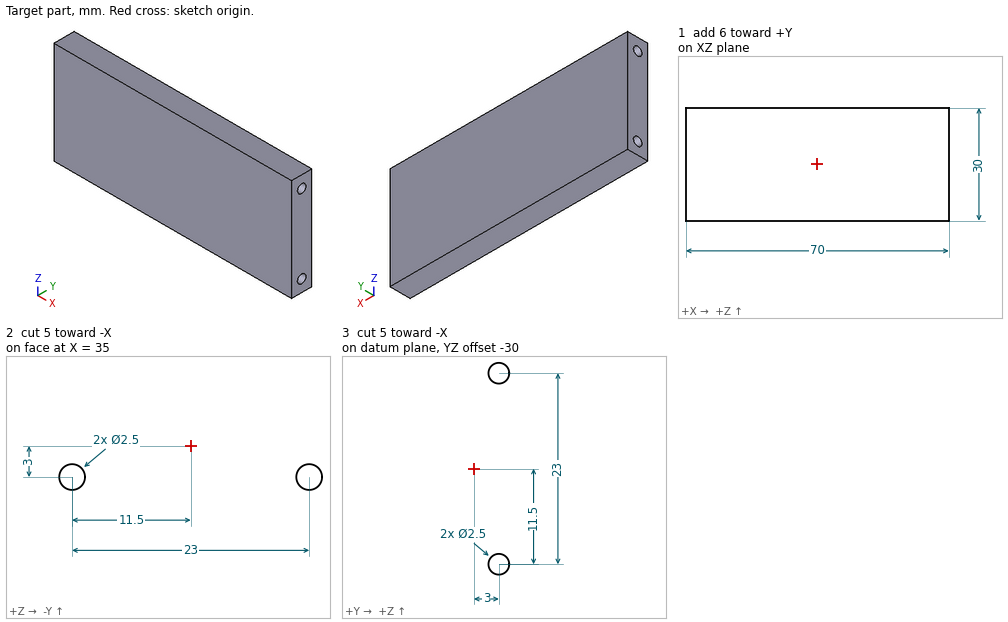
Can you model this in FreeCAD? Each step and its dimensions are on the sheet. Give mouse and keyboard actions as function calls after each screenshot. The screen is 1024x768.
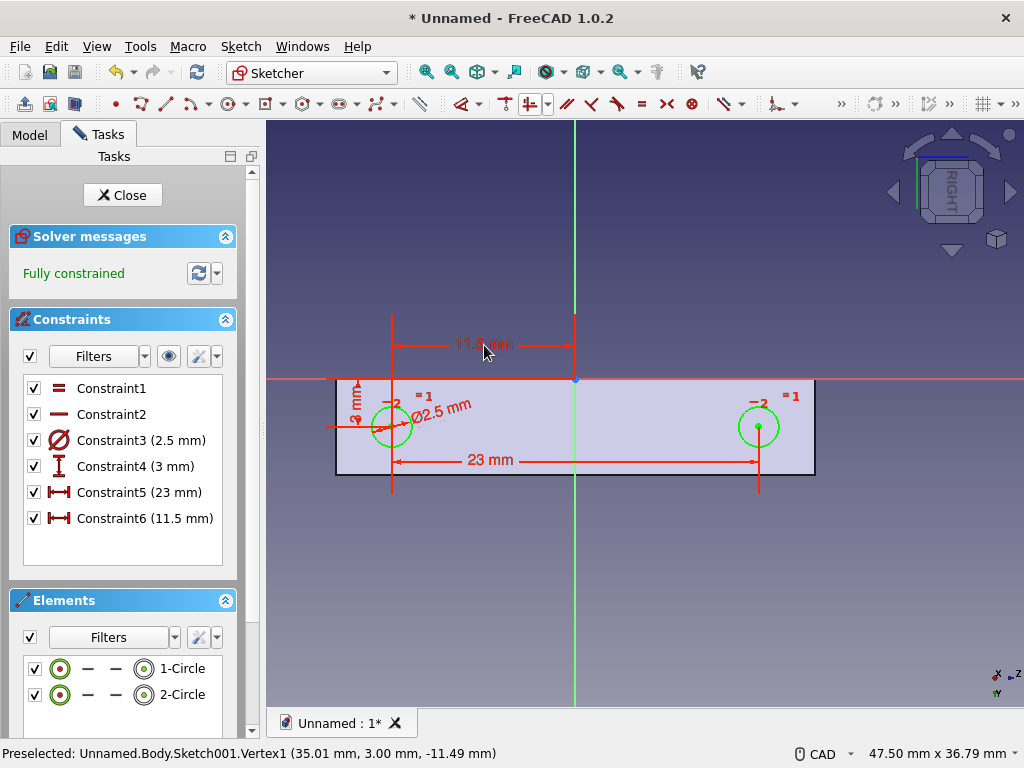
click(123, 195)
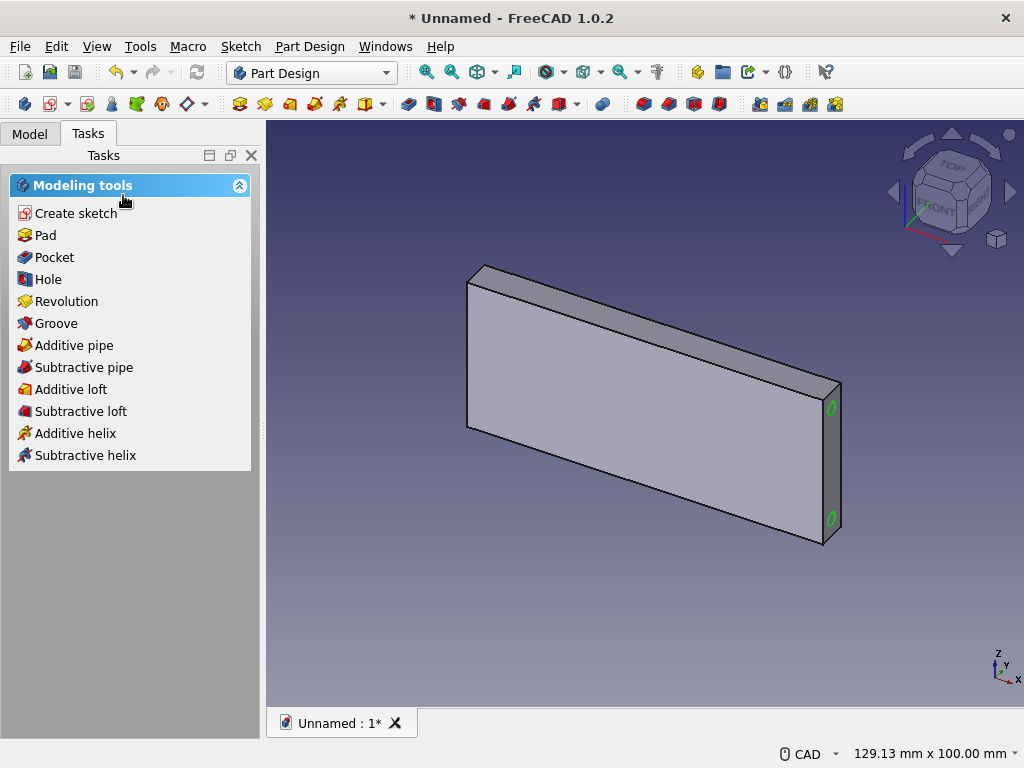
click(409, 104)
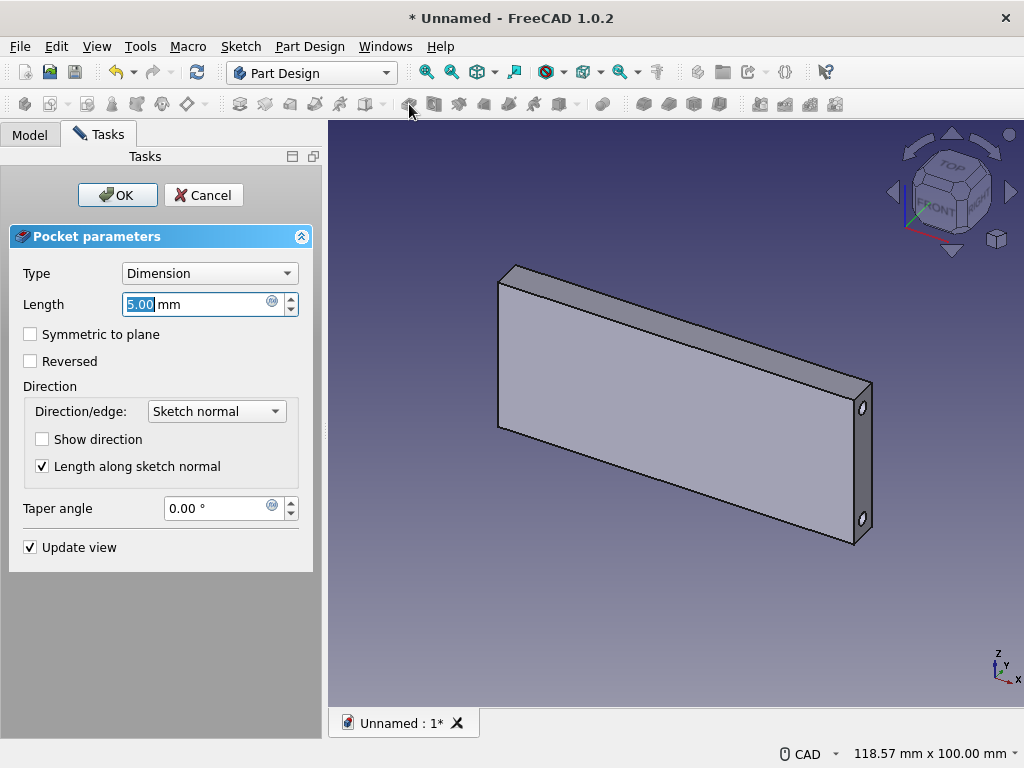
text(5)
key(Tab)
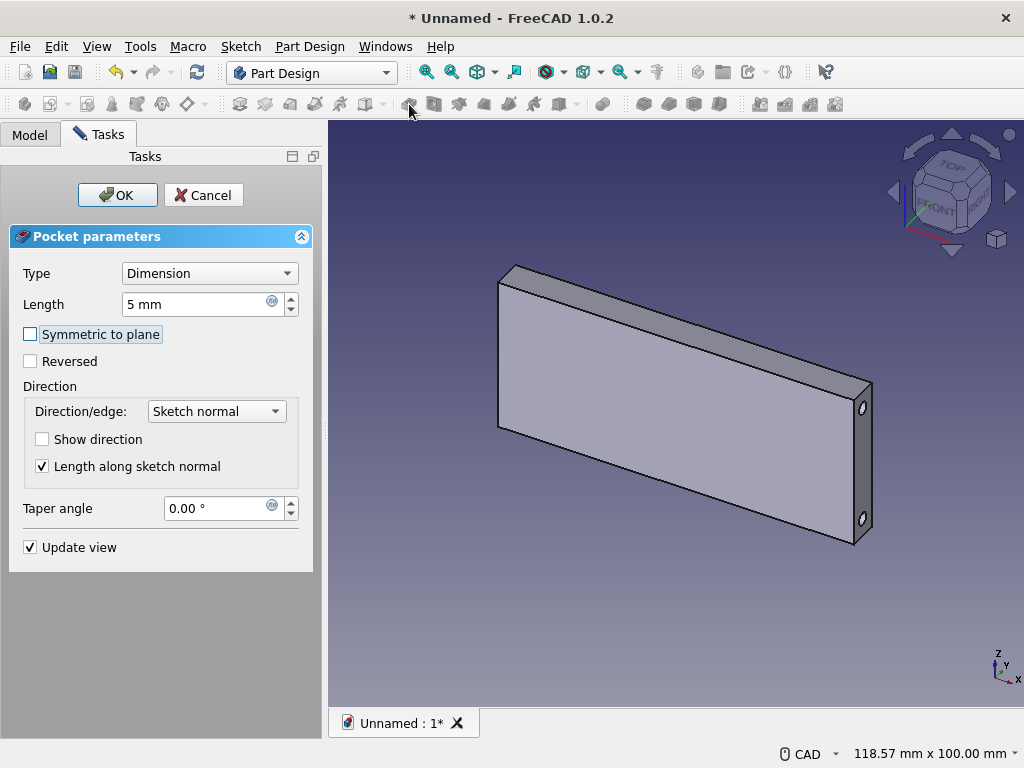
click(118, 195)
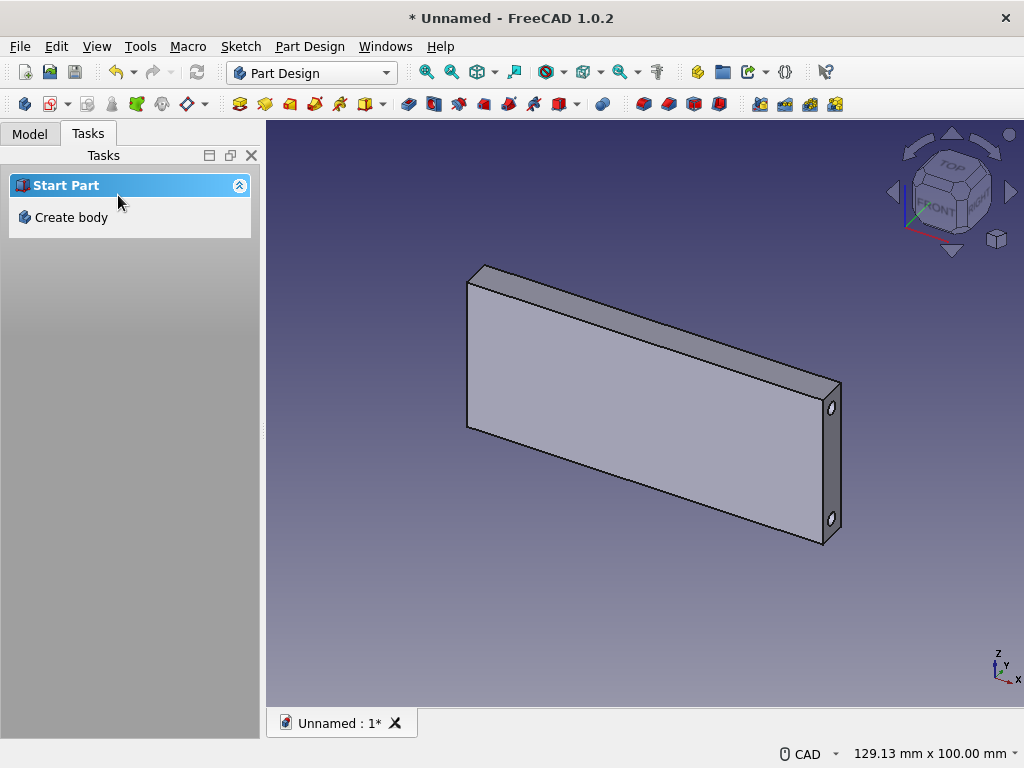
click(30, 134)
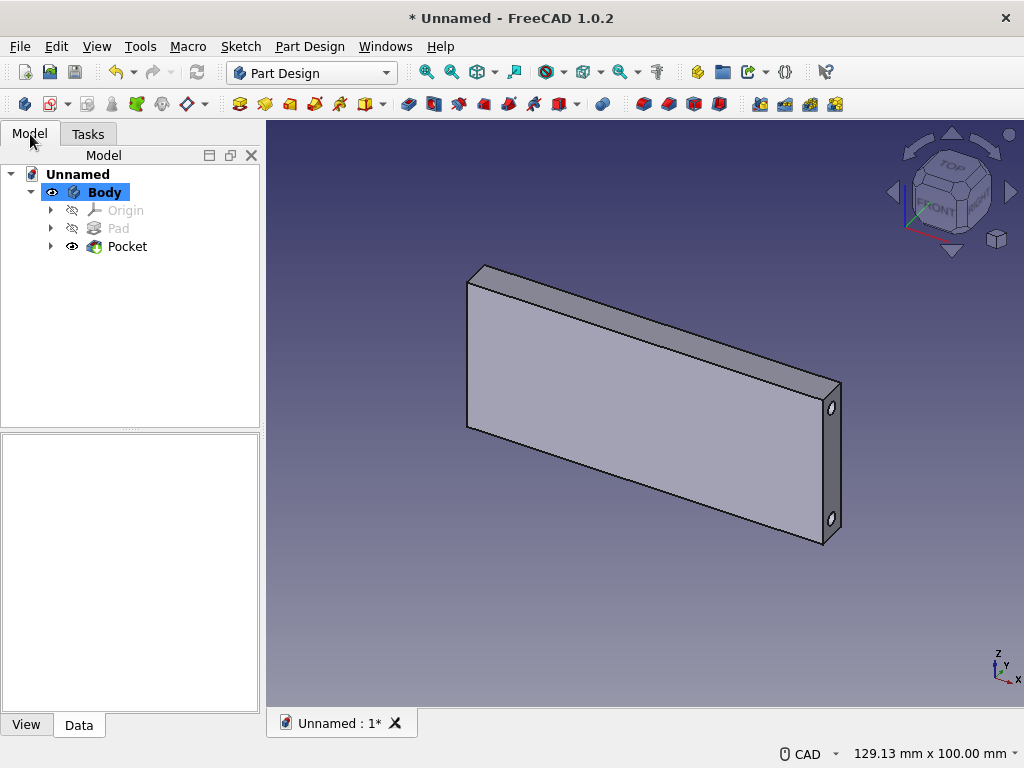
click(51, 210)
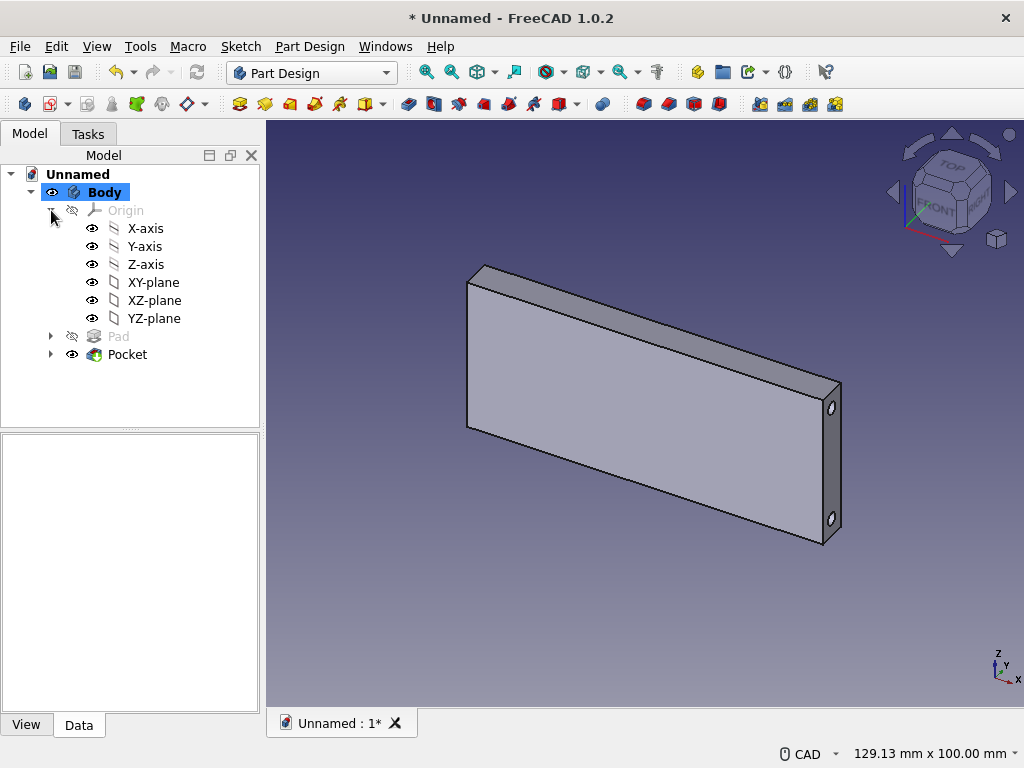
click(137, 318)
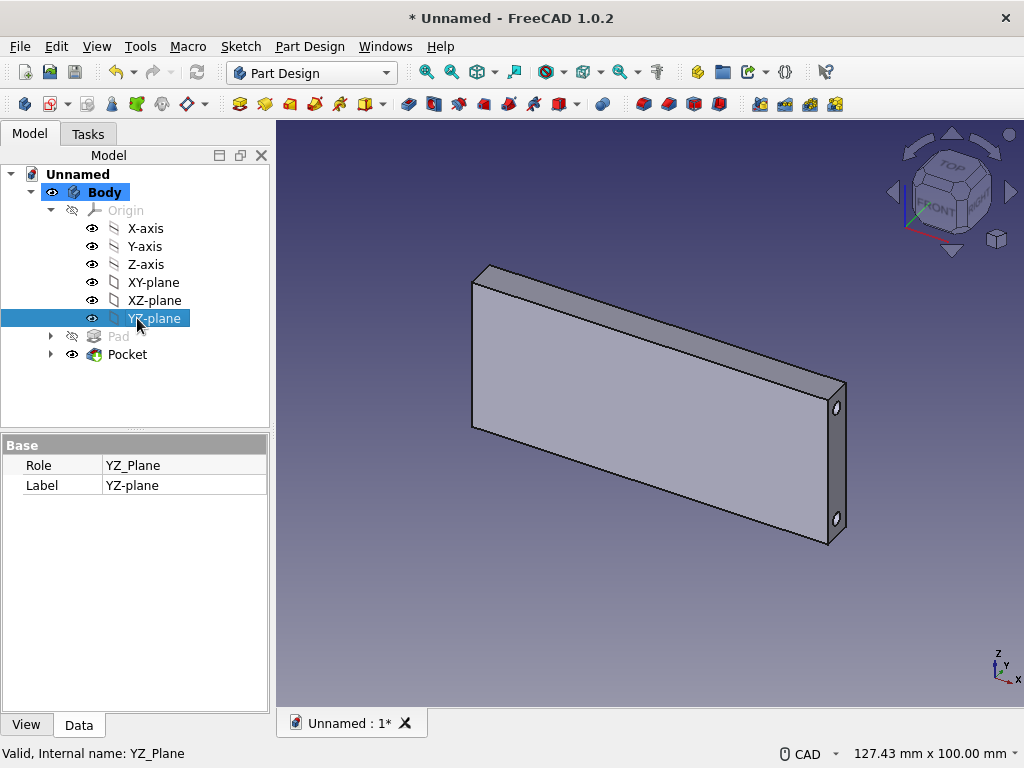
click(186, 104)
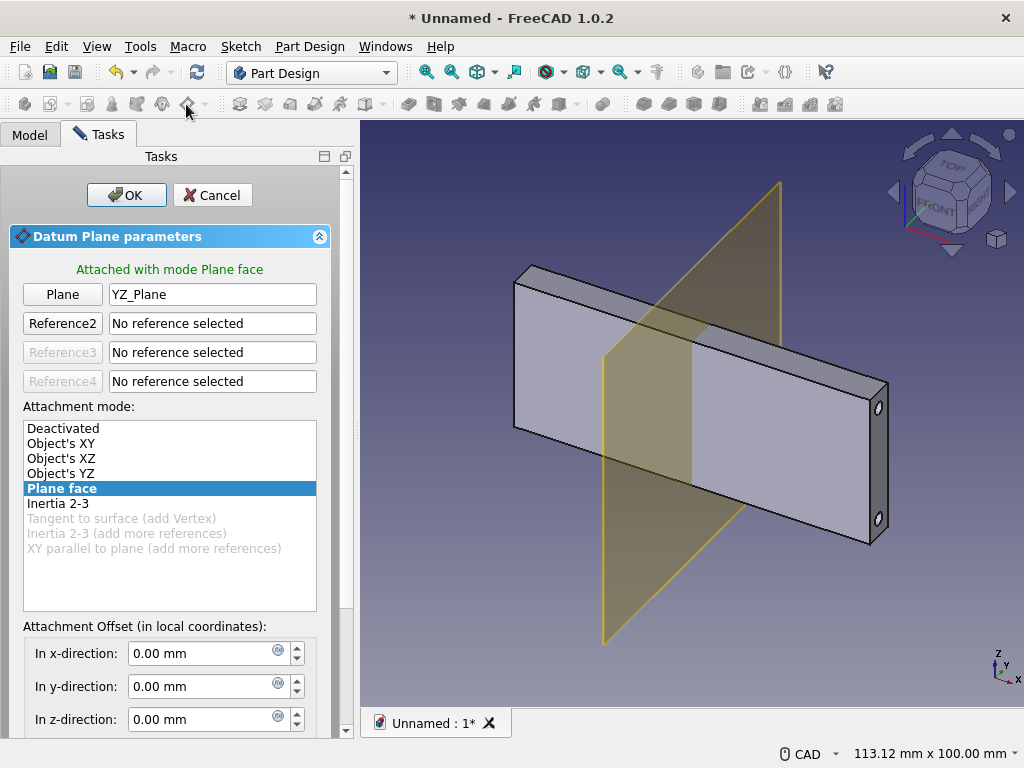
triple_click(210, 720)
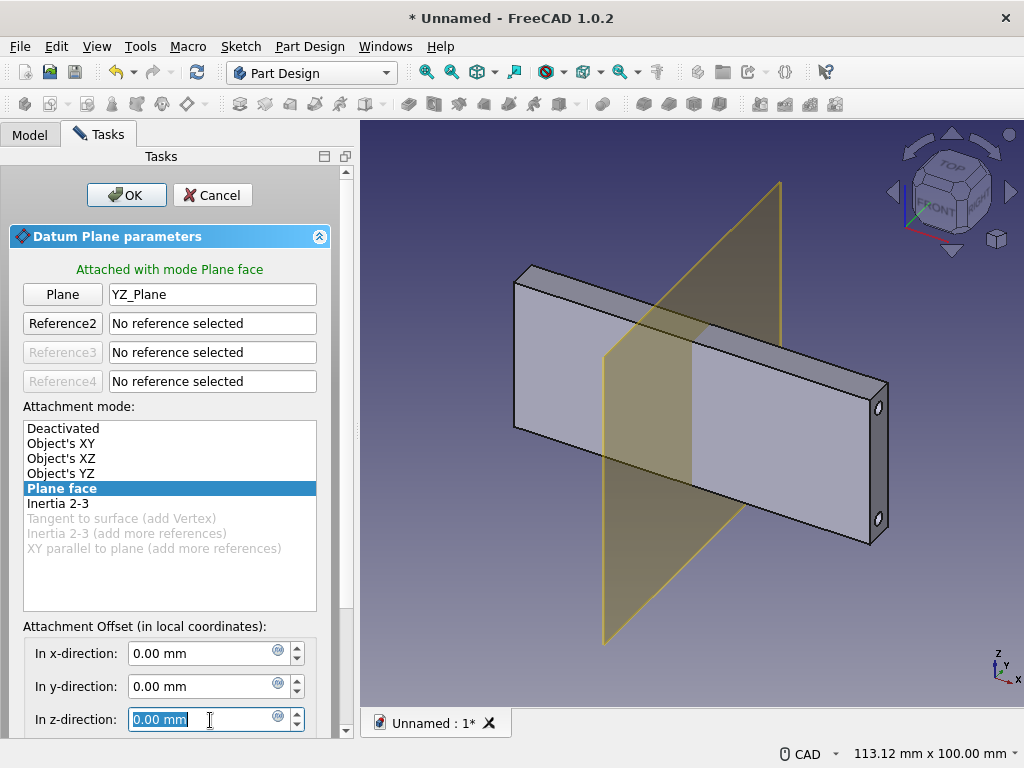
text(-30)
key(Tab)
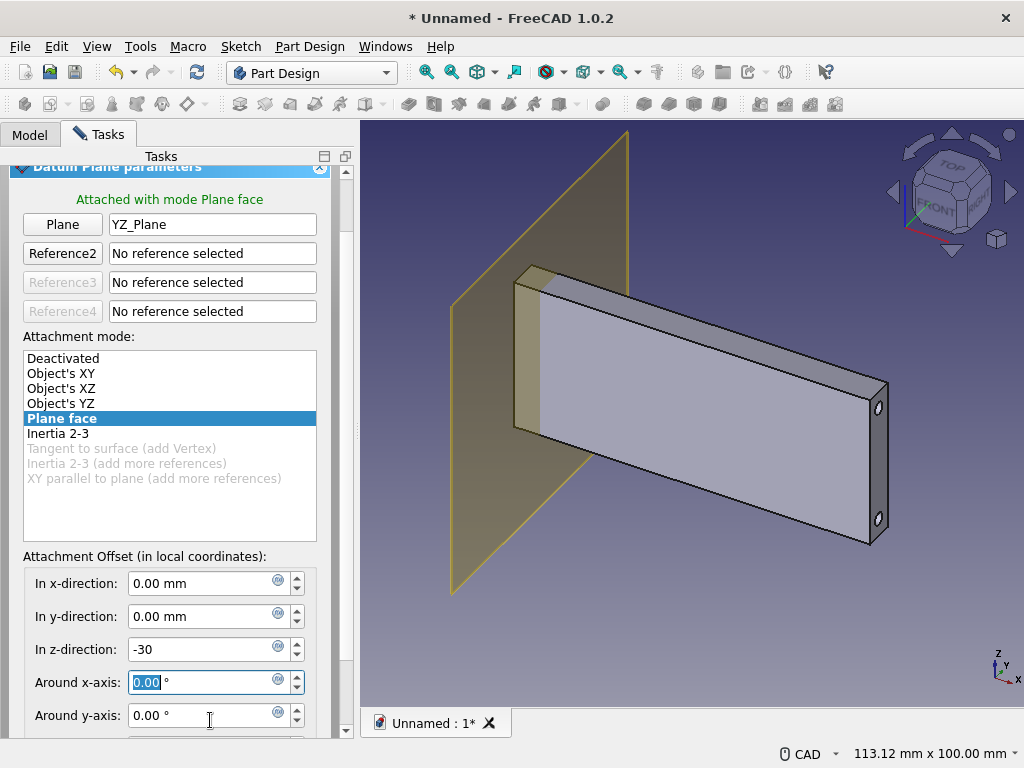
scroll(346, 452, up, 2)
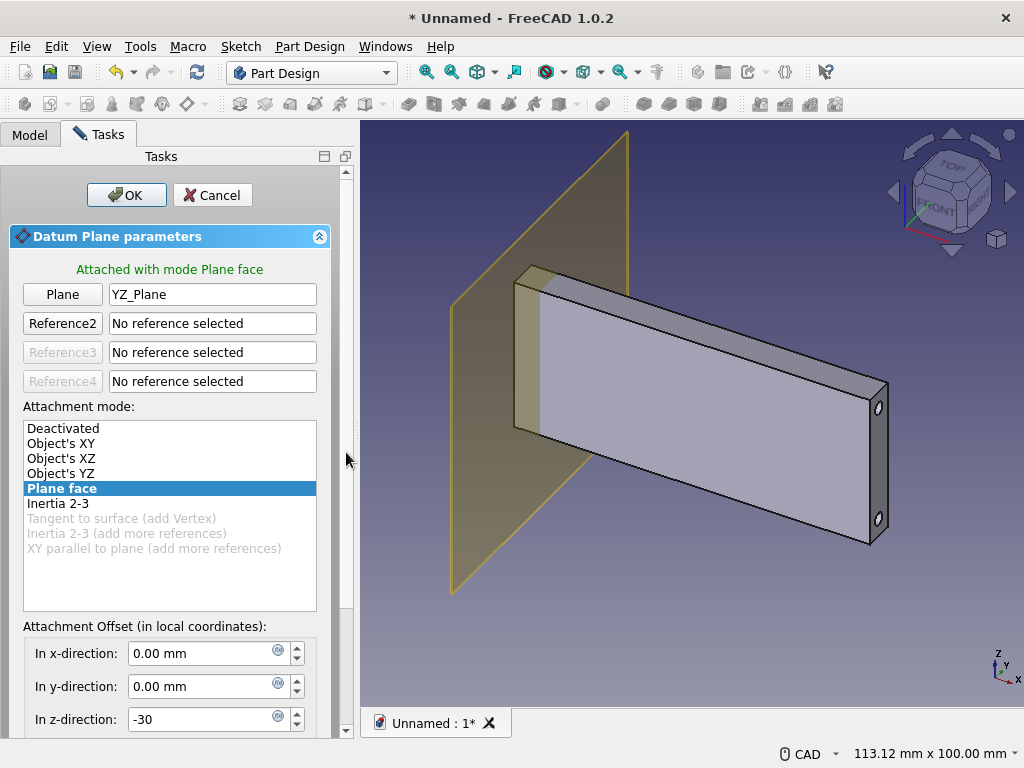
click(127, 195)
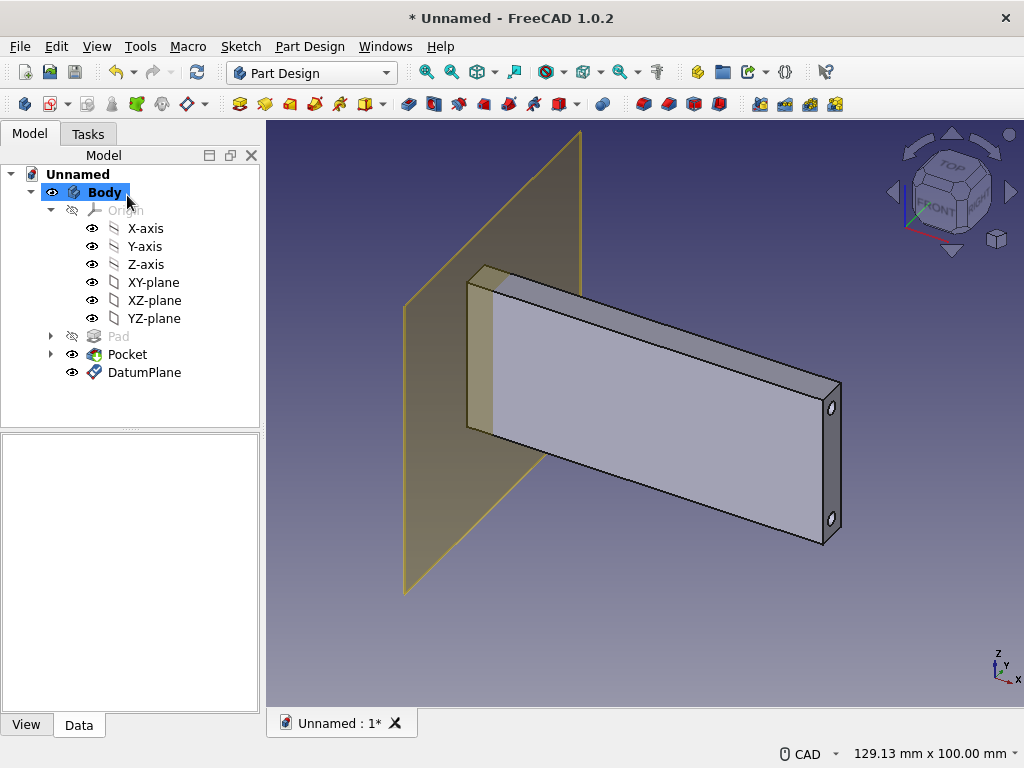
click(117, 372)